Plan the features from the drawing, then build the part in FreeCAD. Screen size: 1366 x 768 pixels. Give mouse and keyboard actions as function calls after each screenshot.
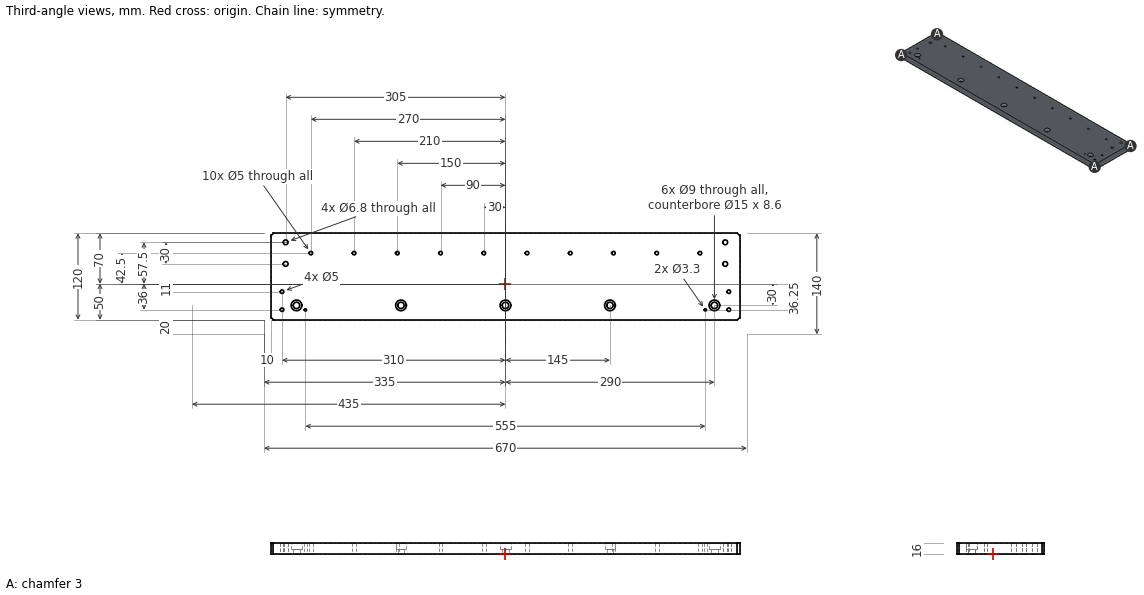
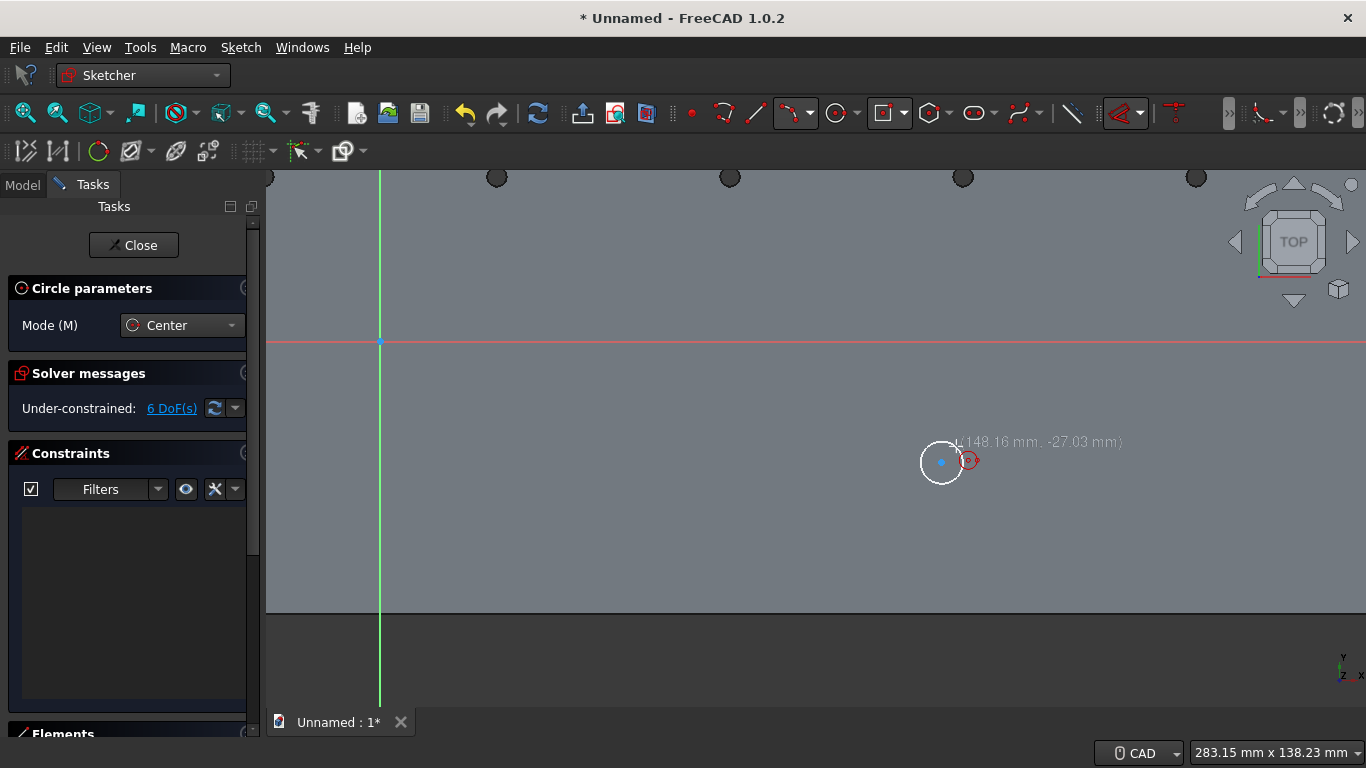
scroll(380, 459, up, 2)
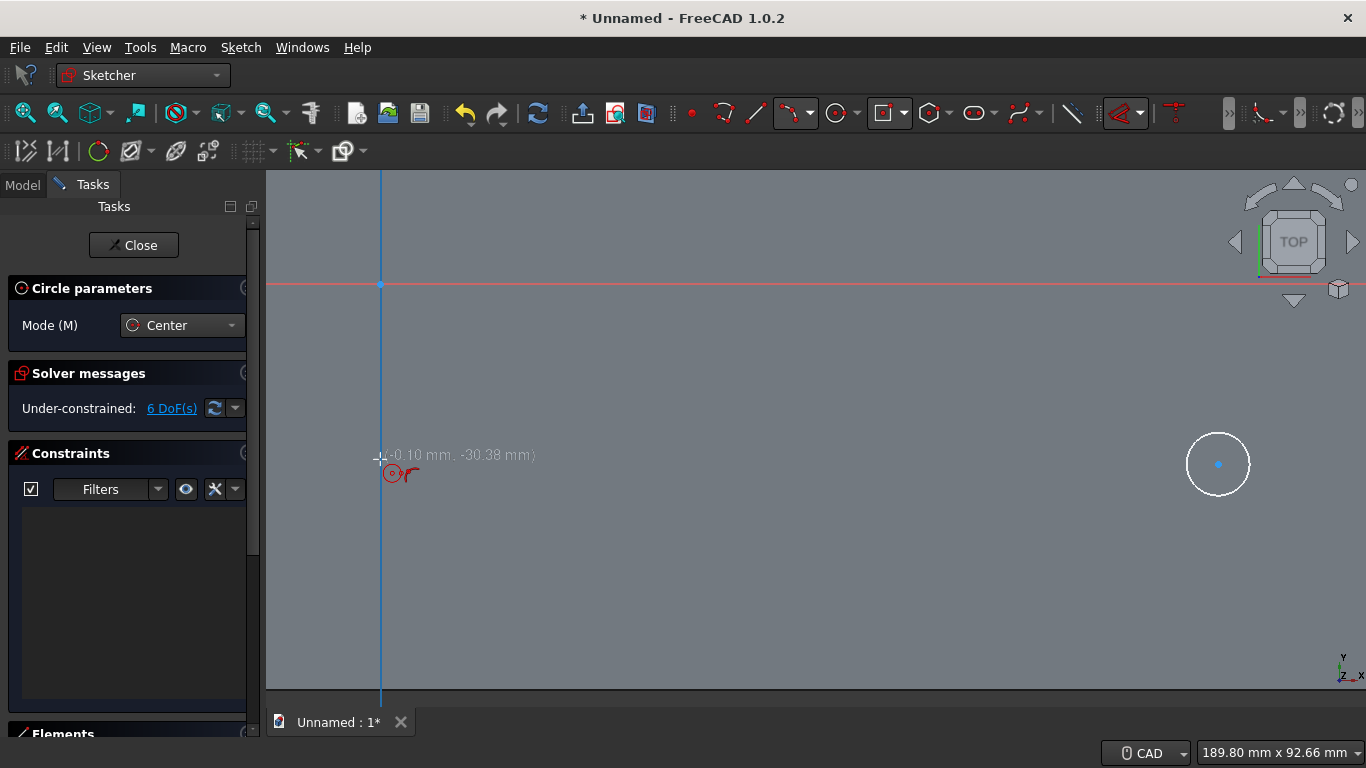
scroll(903, 449, down, 9)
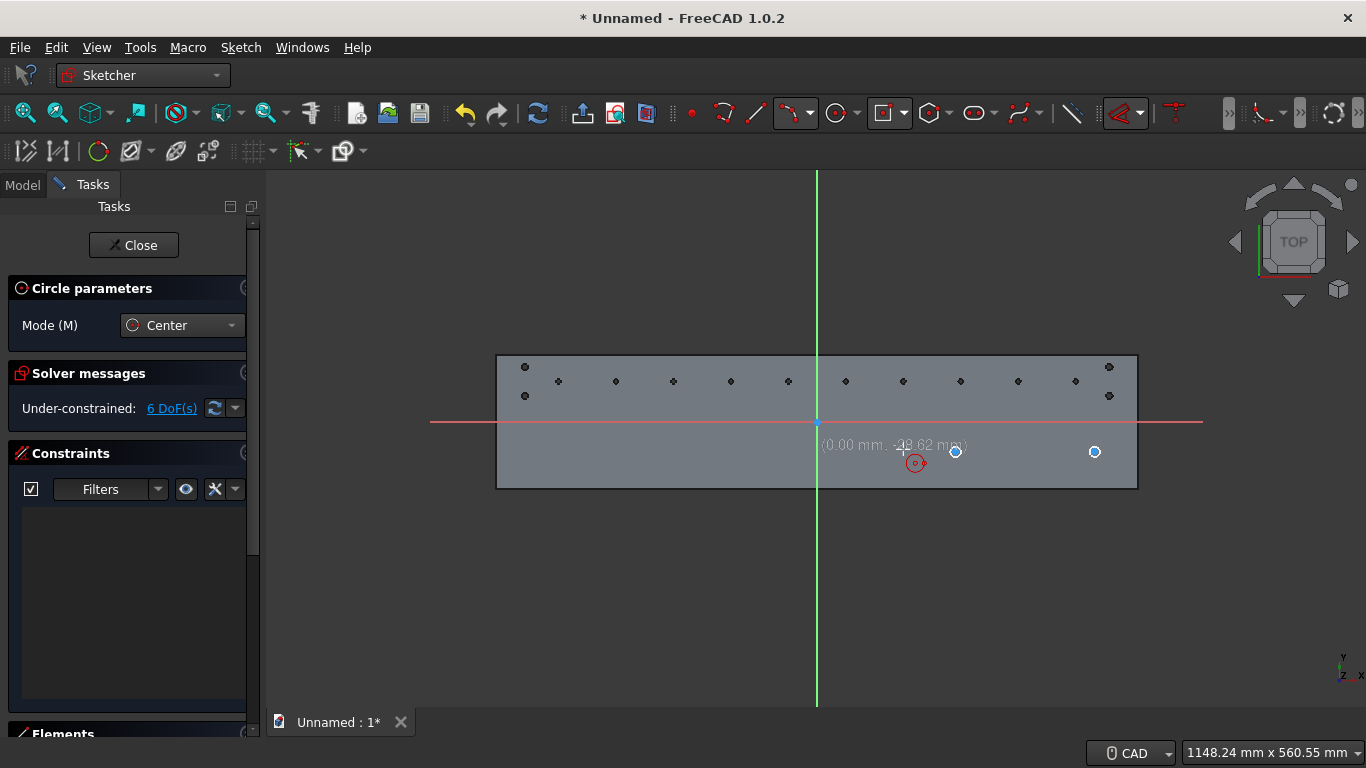
click(817, 451)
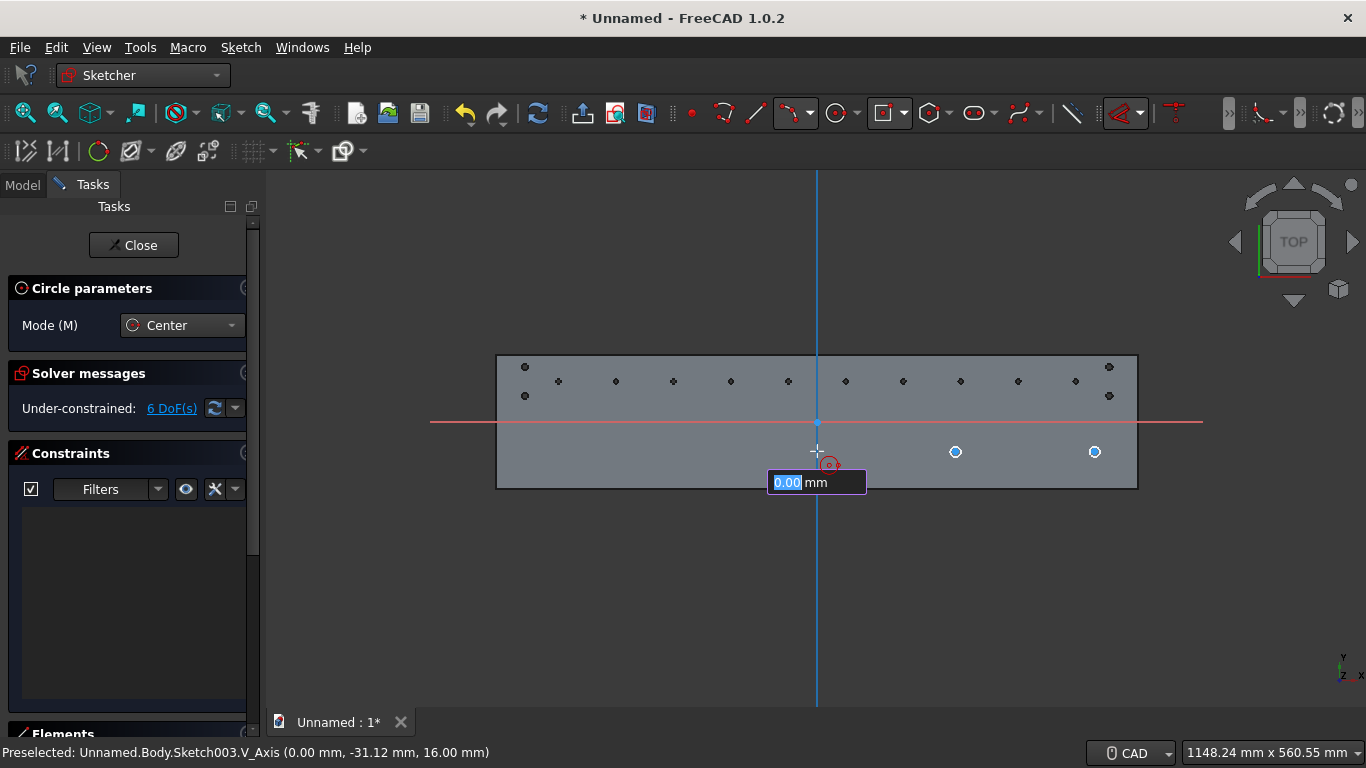
scroll(821, 449, up, 7)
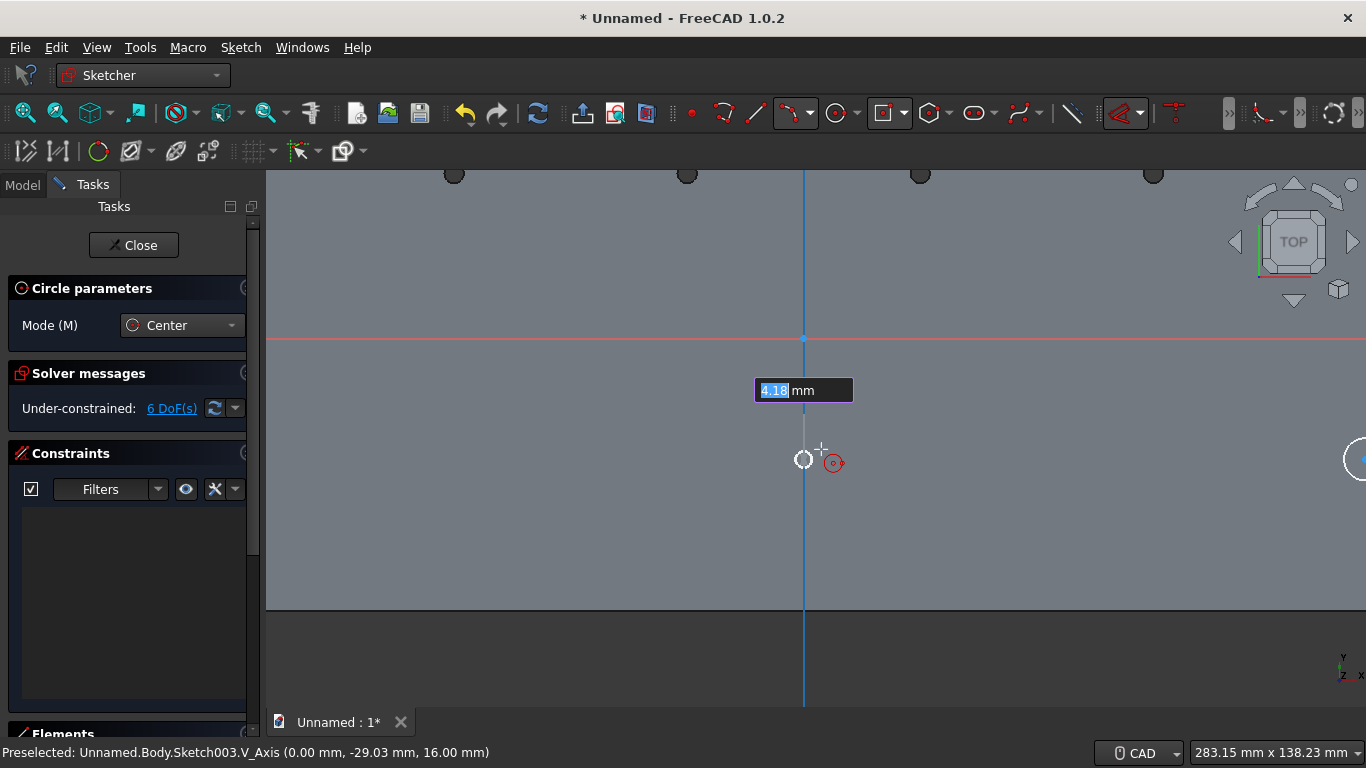
click(820, 449)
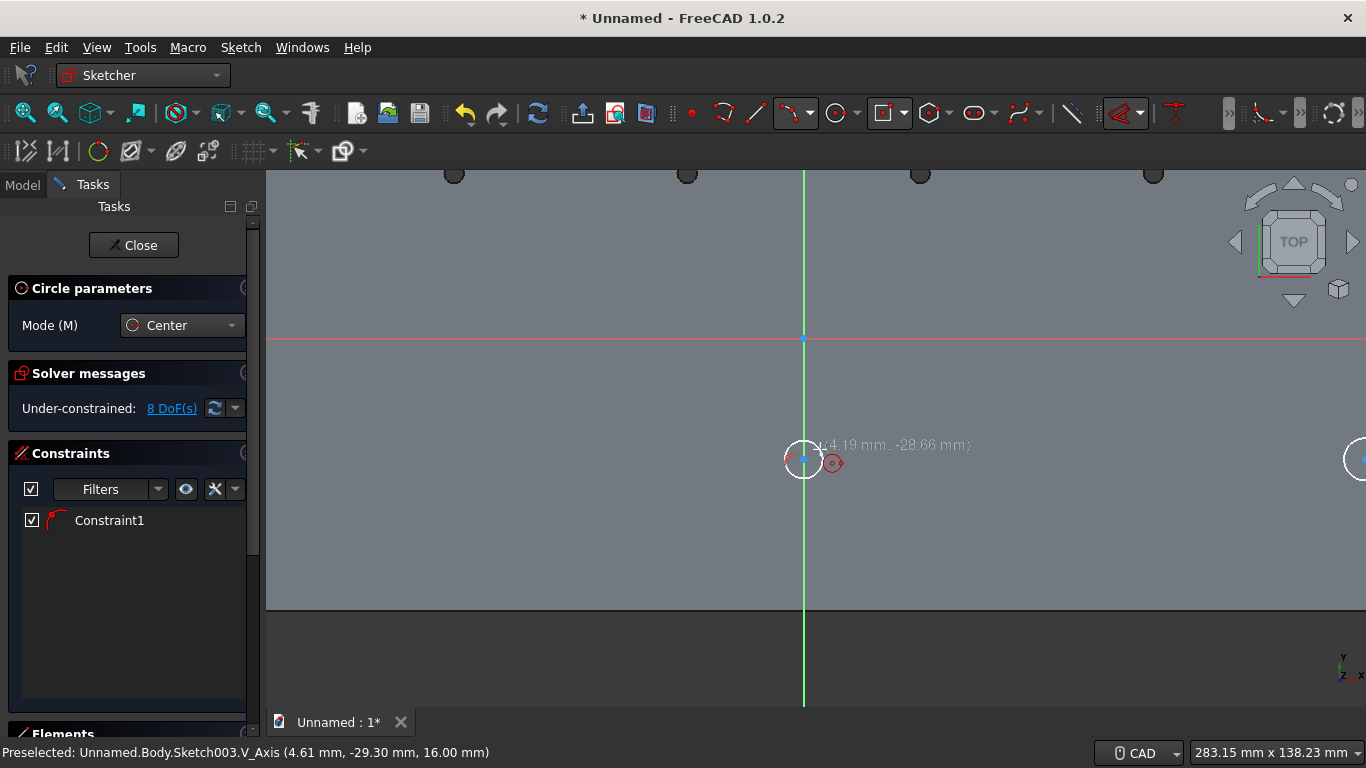
scroll(821, 449, down, 7)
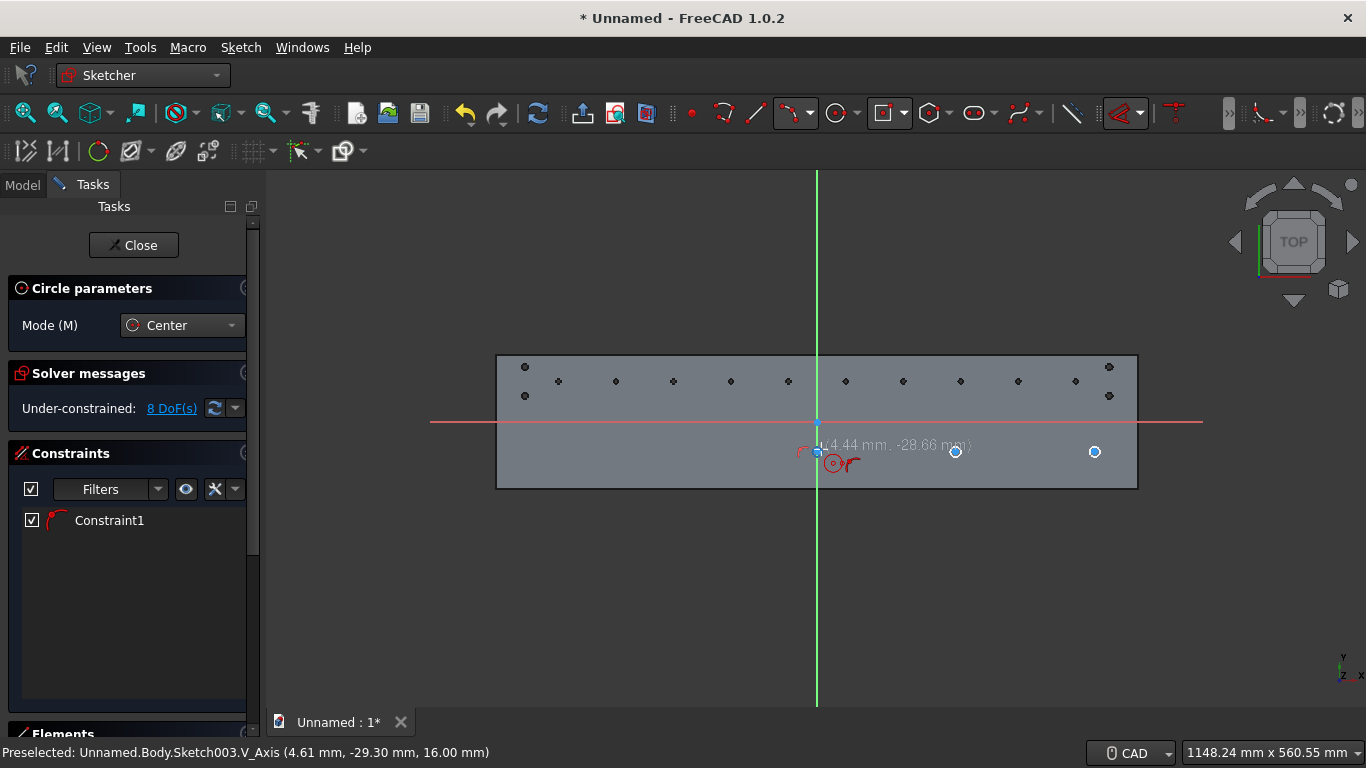
scroll(678, 451, up, 9)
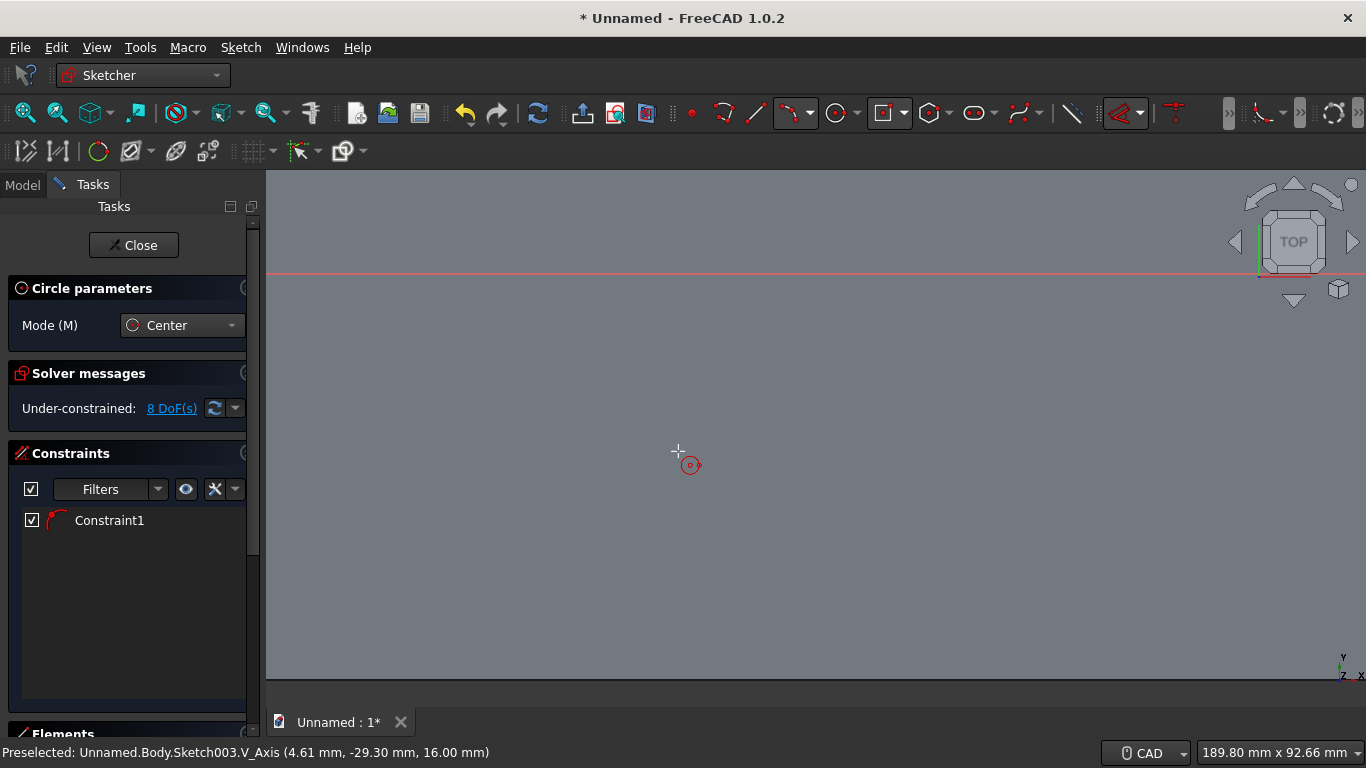
scroll(678, 451, down, 9)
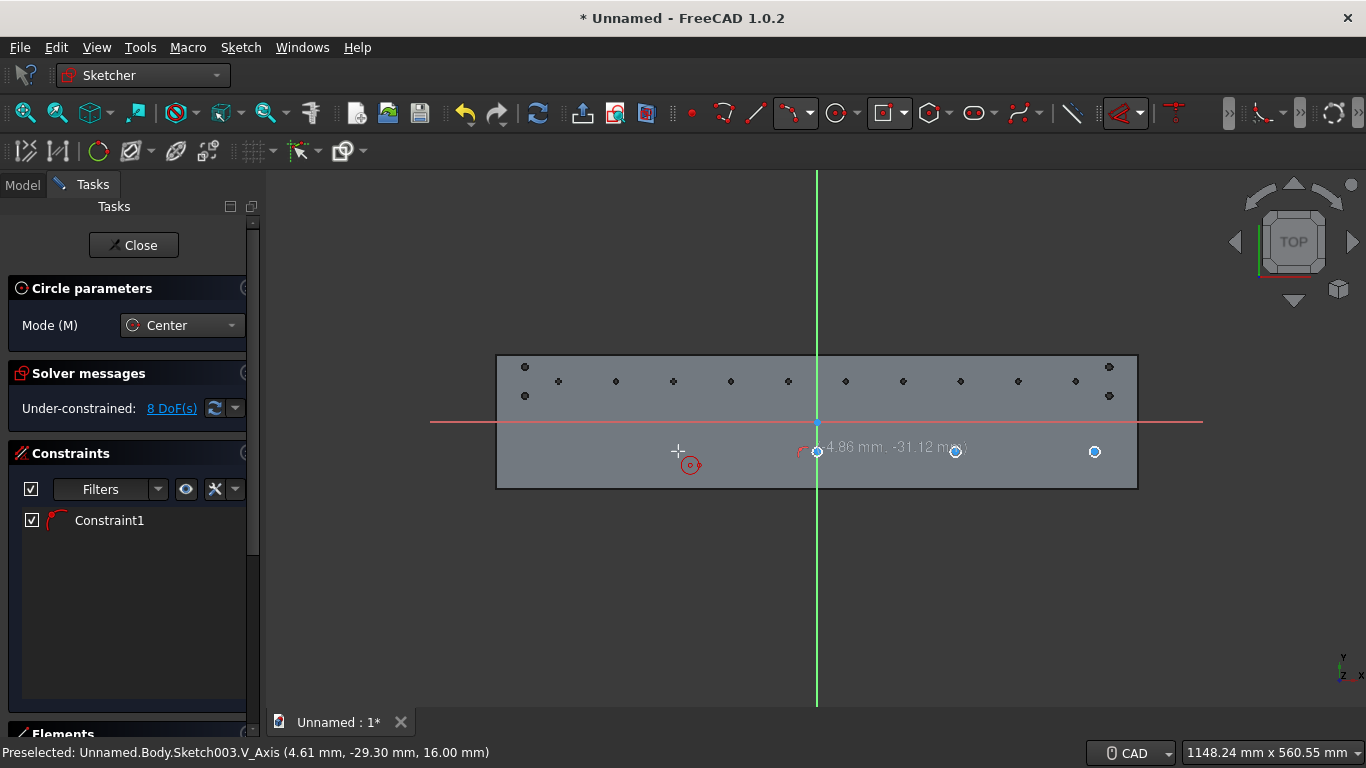
click(678, 451)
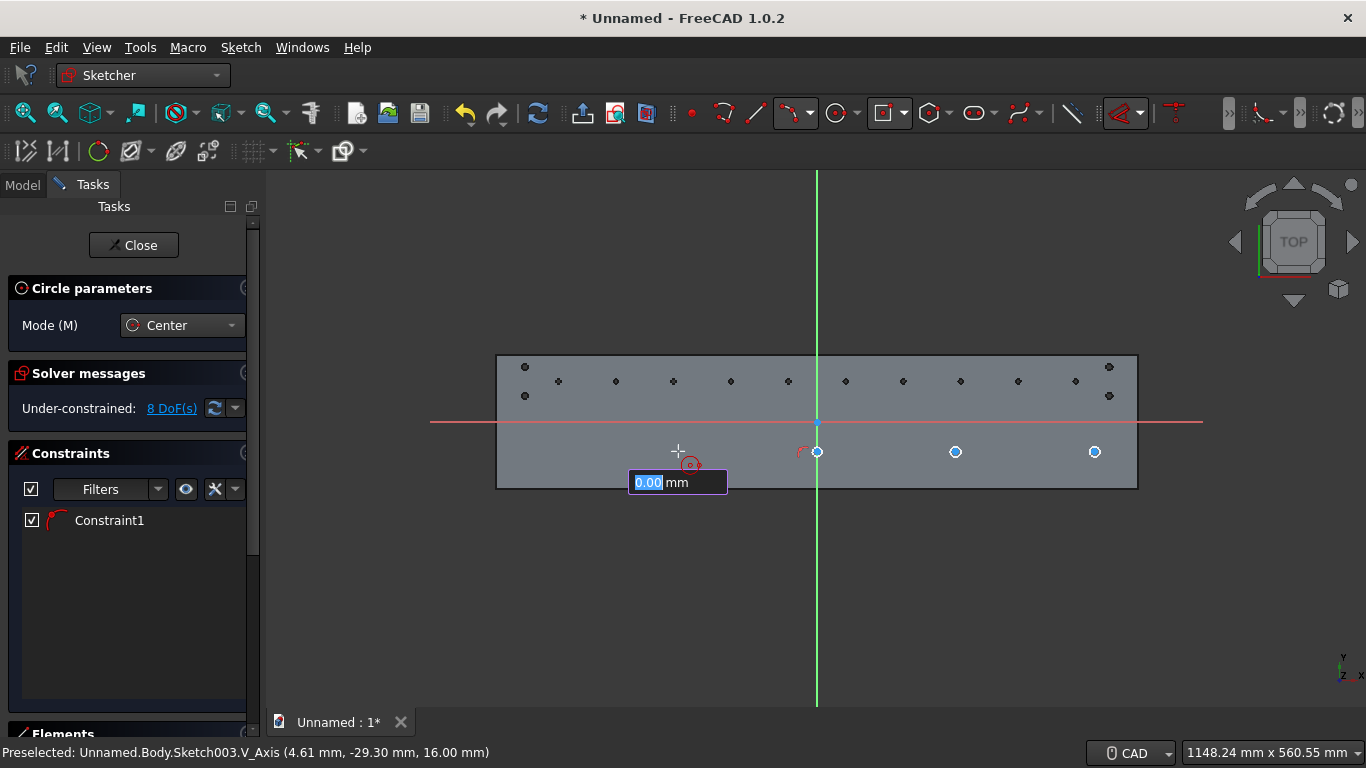
scroll(681, 448, up, 7)